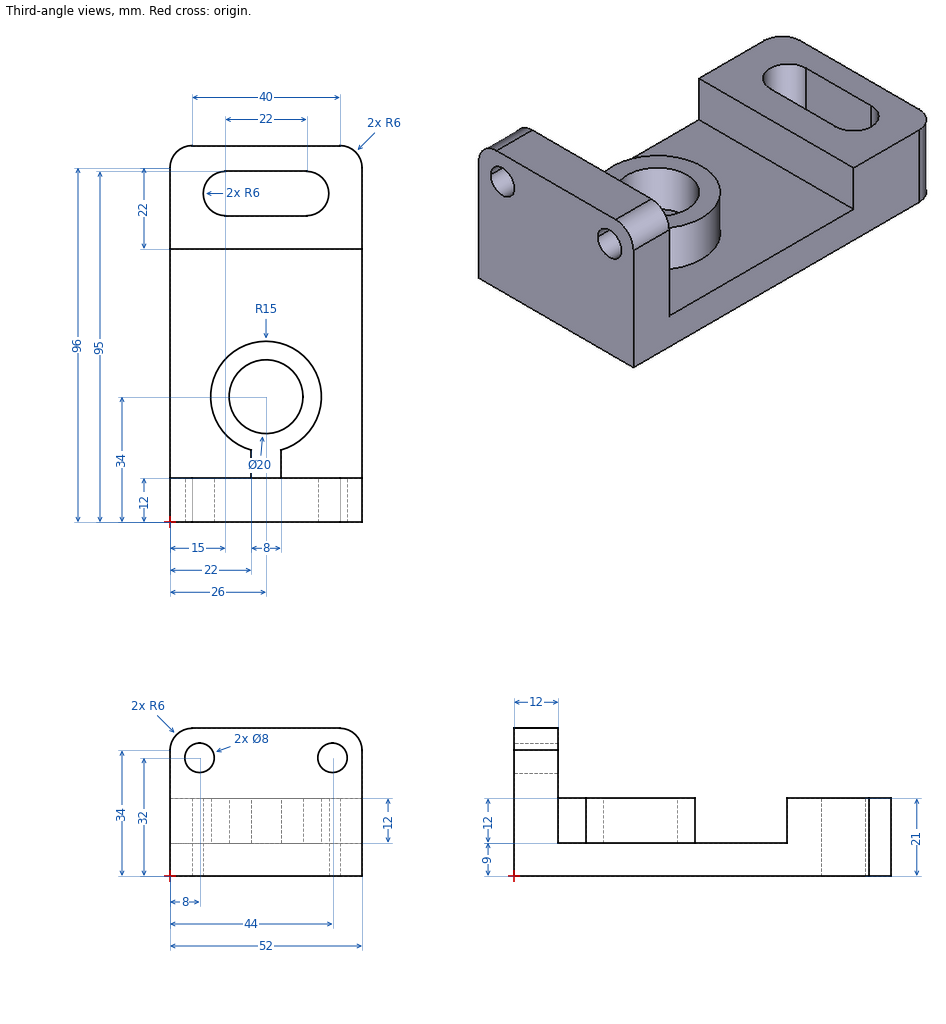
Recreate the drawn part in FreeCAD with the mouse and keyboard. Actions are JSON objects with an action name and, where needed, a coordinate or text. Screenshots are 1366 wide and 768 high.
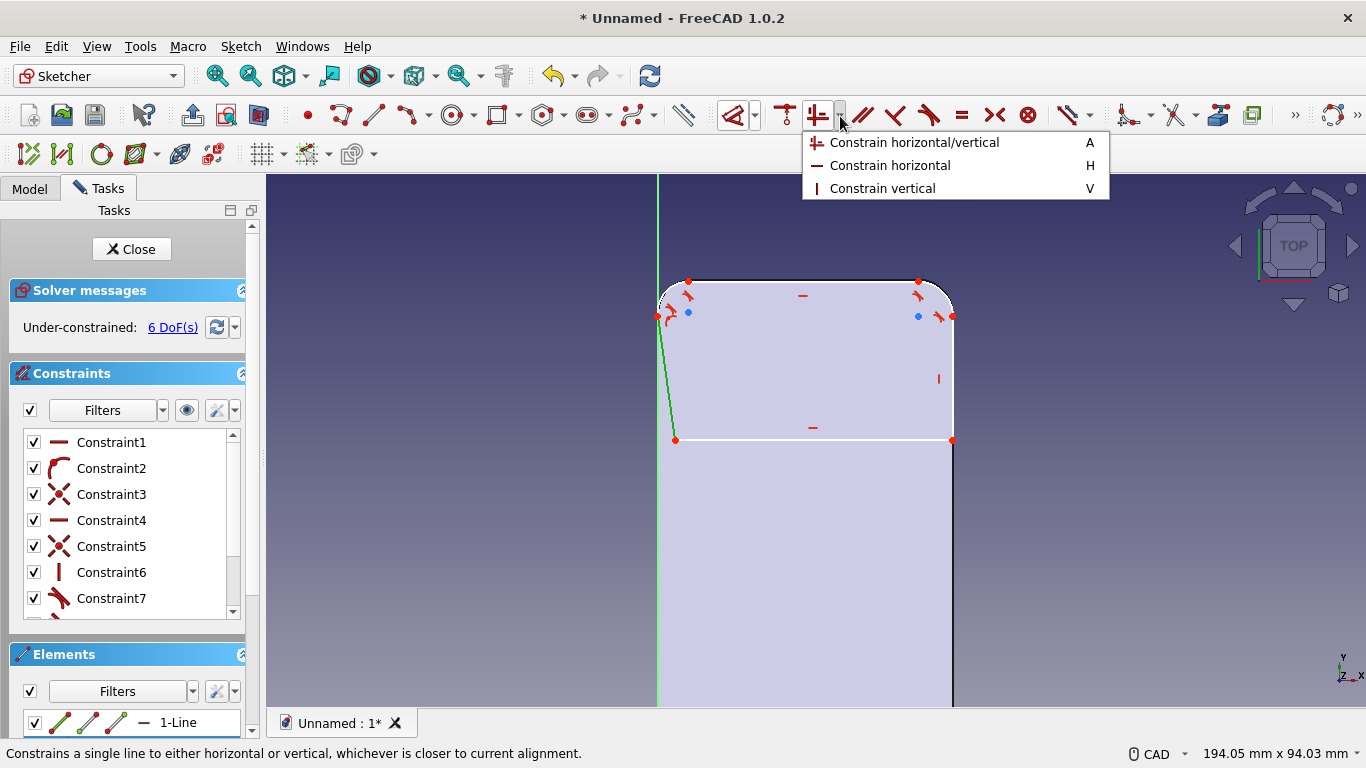
{"action": "left_click", "coordinate": [956, 188]}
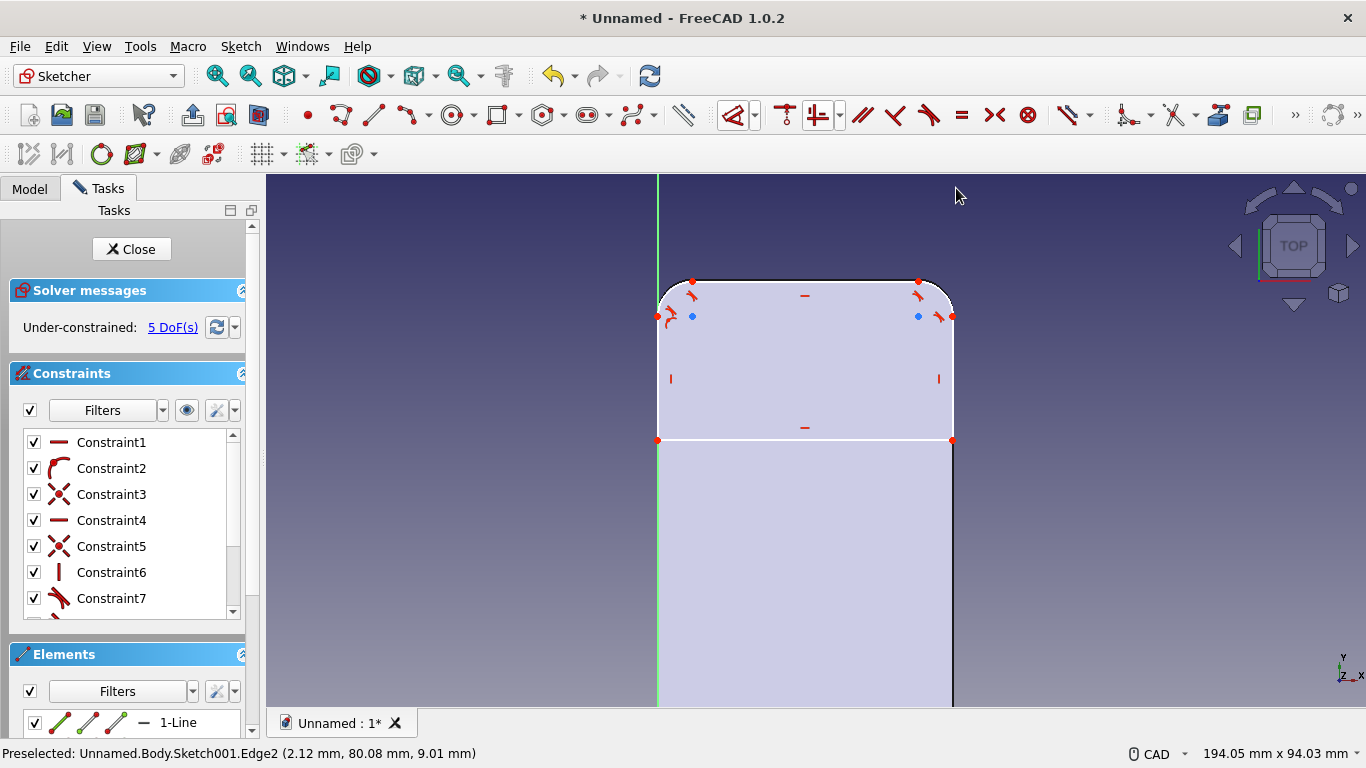
{"action": "left_click", "coordinate": [677, 286]}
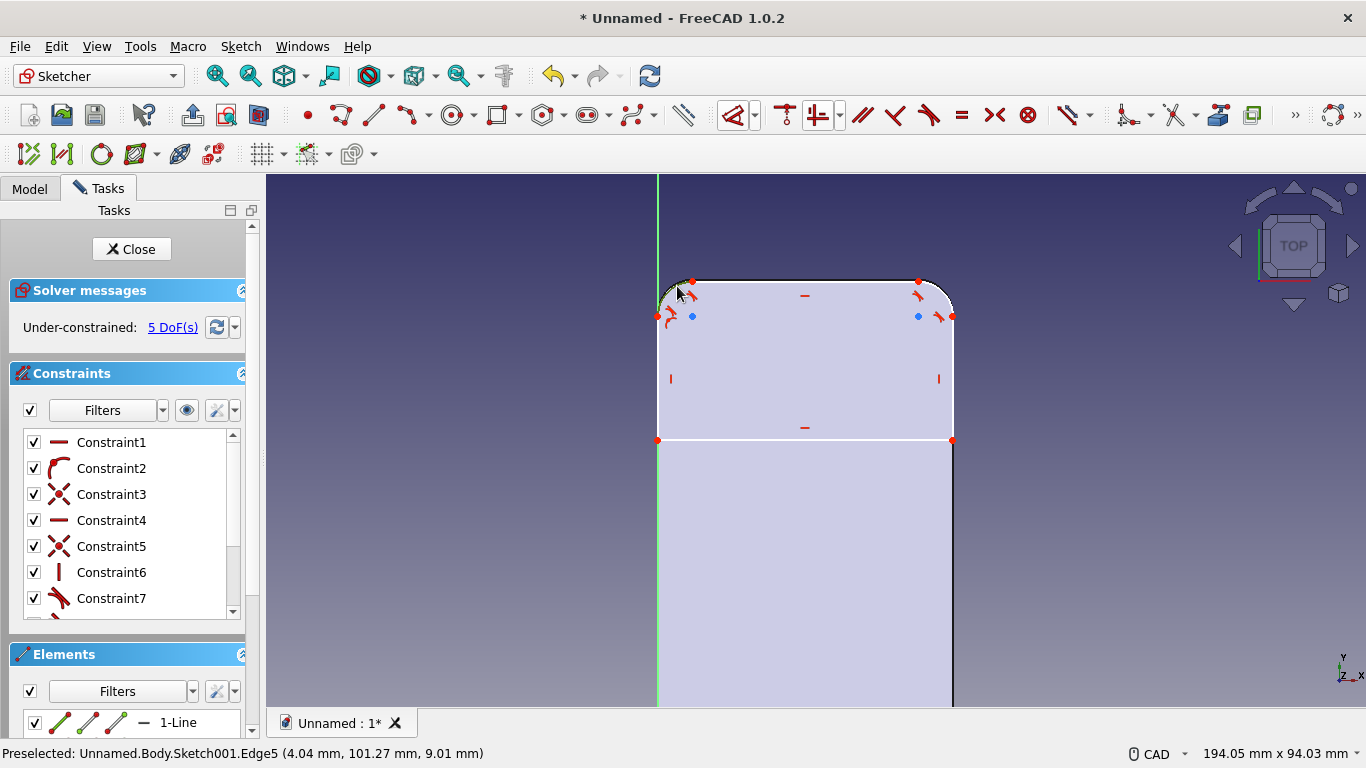
{"action": "left_click", "coordinate": [949, 301]}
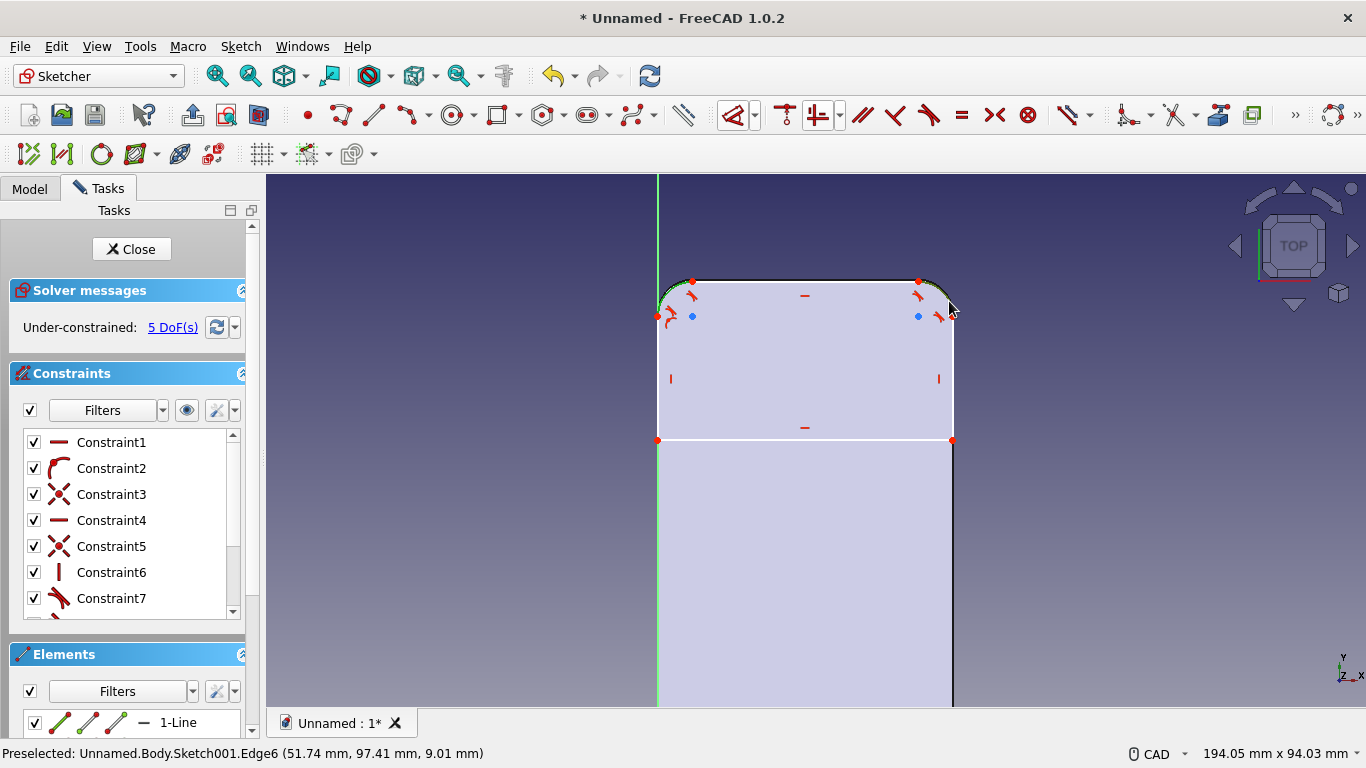
{"action": "left_click", "coordinate": [962, 116]}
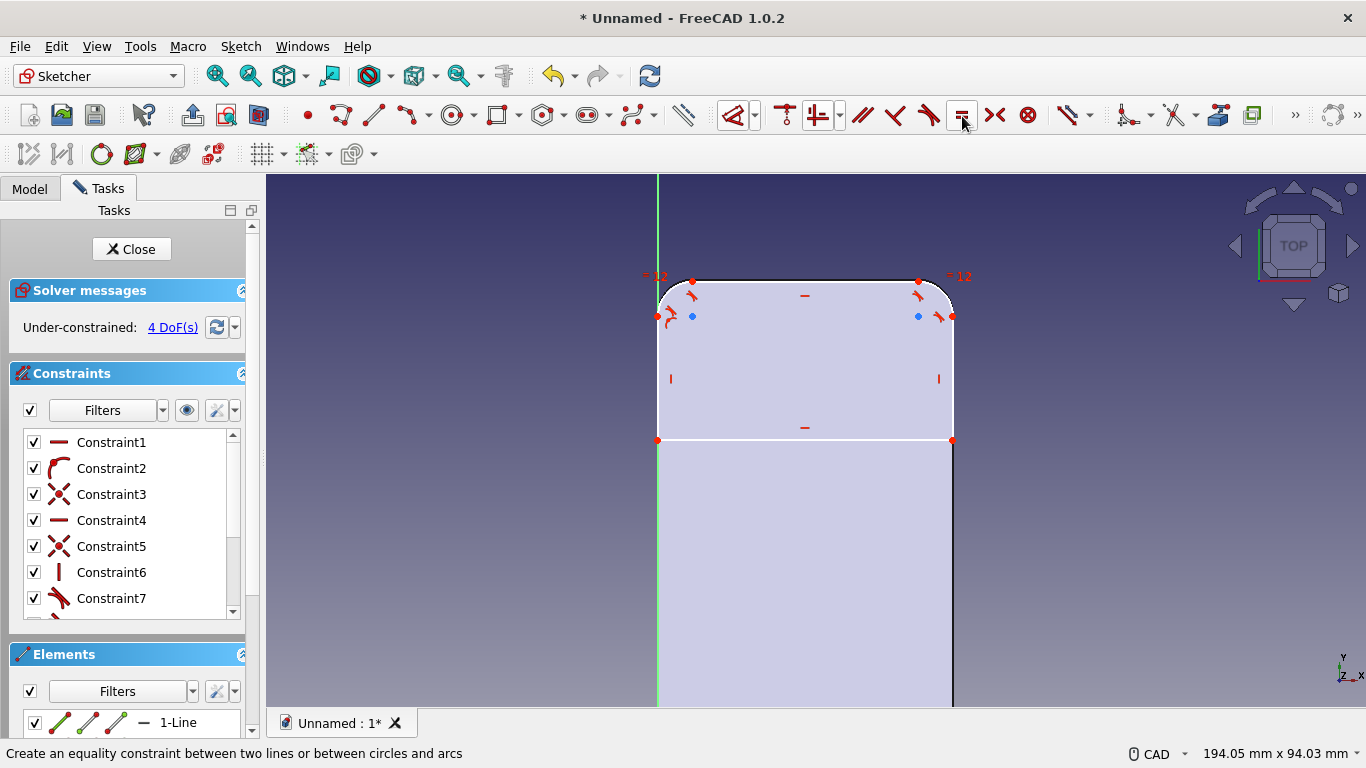
{"action": "left_click", "coordinate": [677, 286]}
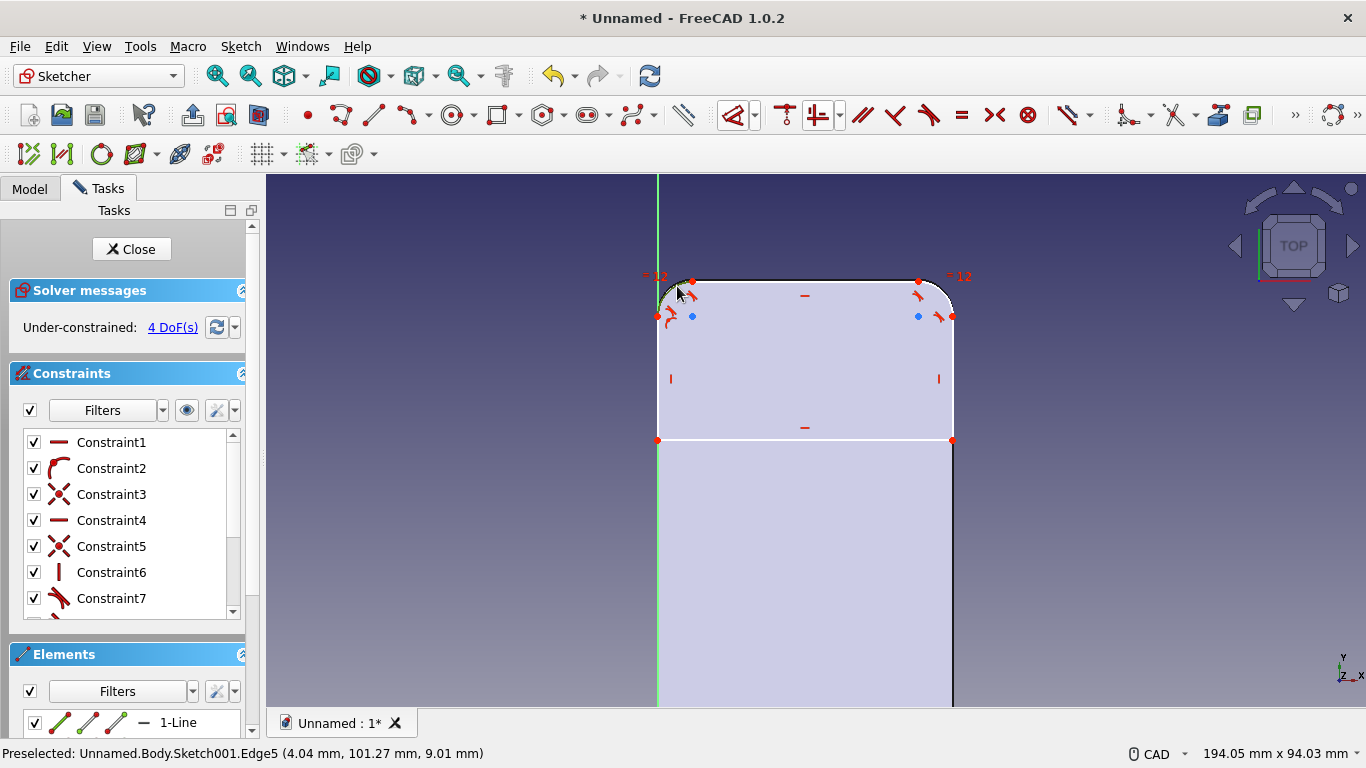
{"action": "key", "text": "k r"}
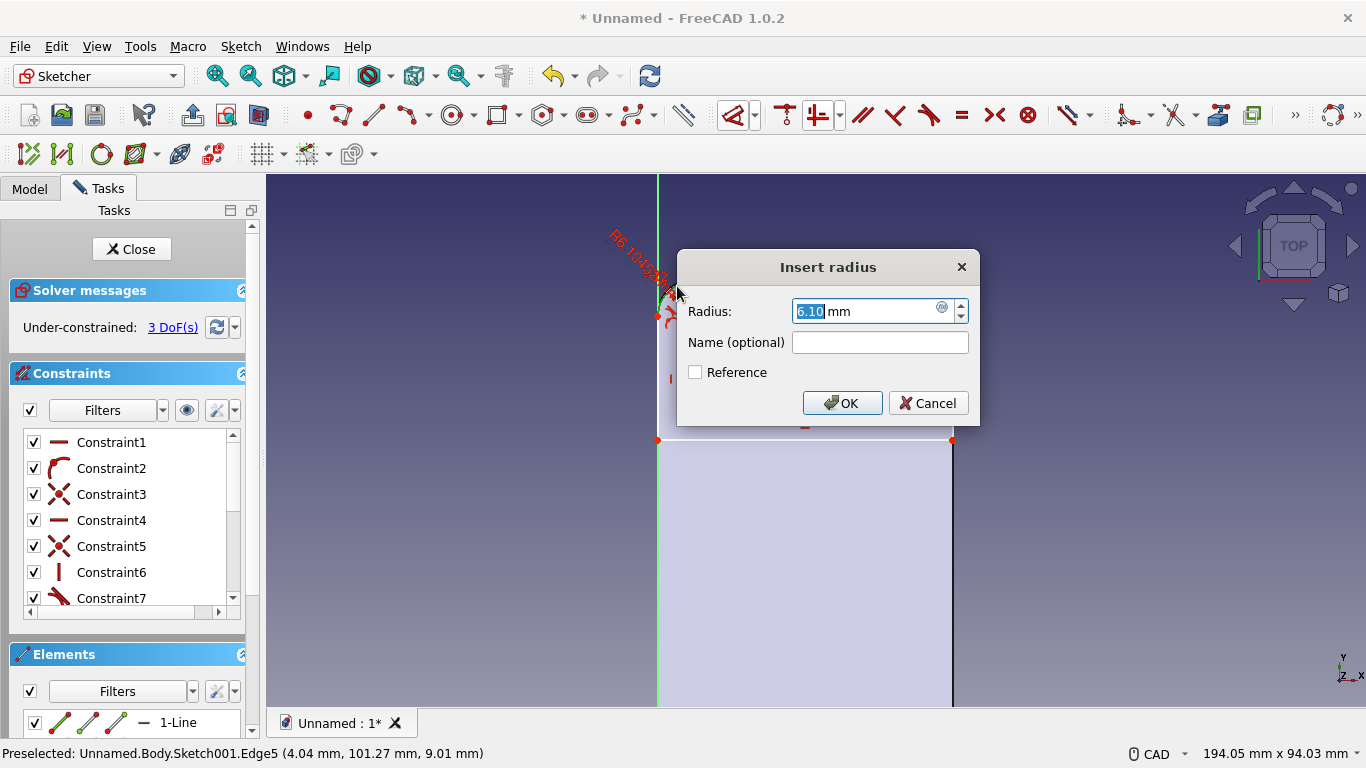
{"action": "type", "text": "6"}
{"action": "key", "text": "Return"}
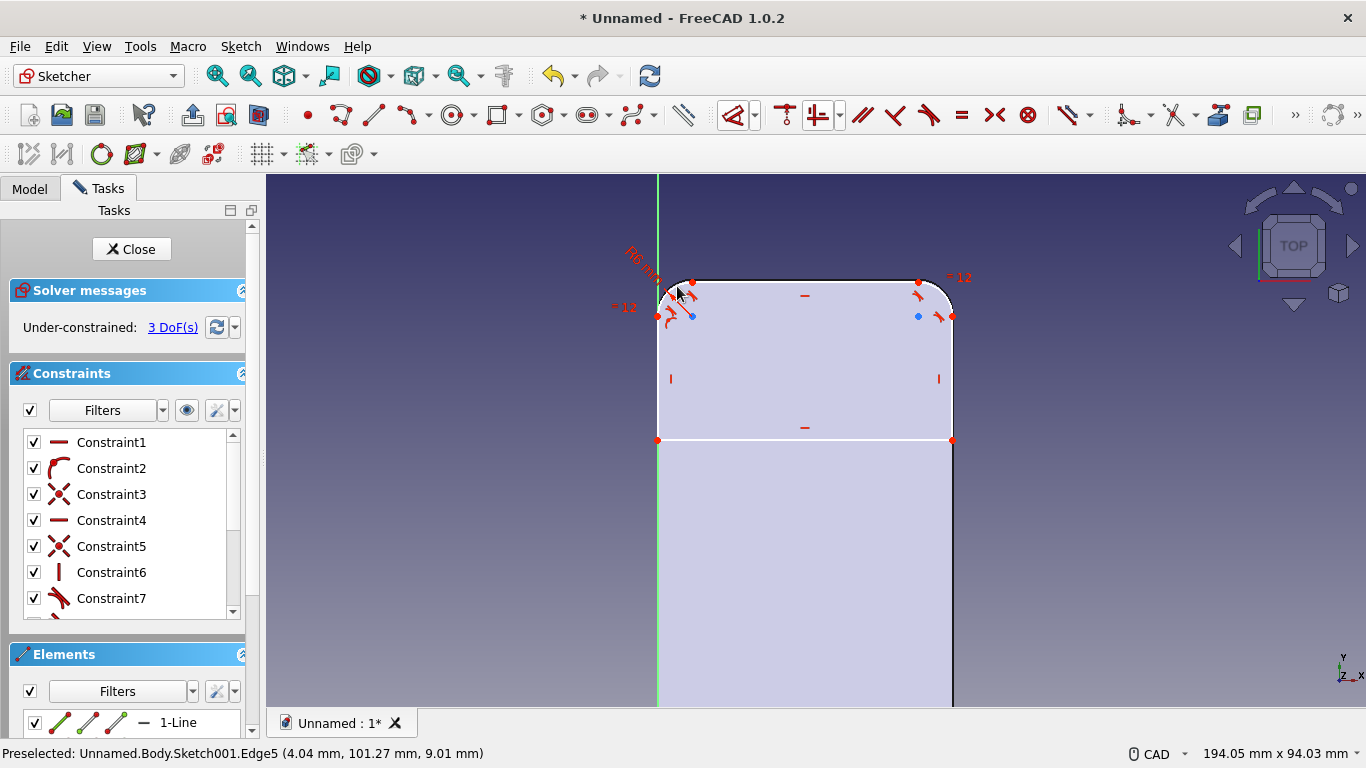
{"action": "left_click", "coordinate": [850, 282]}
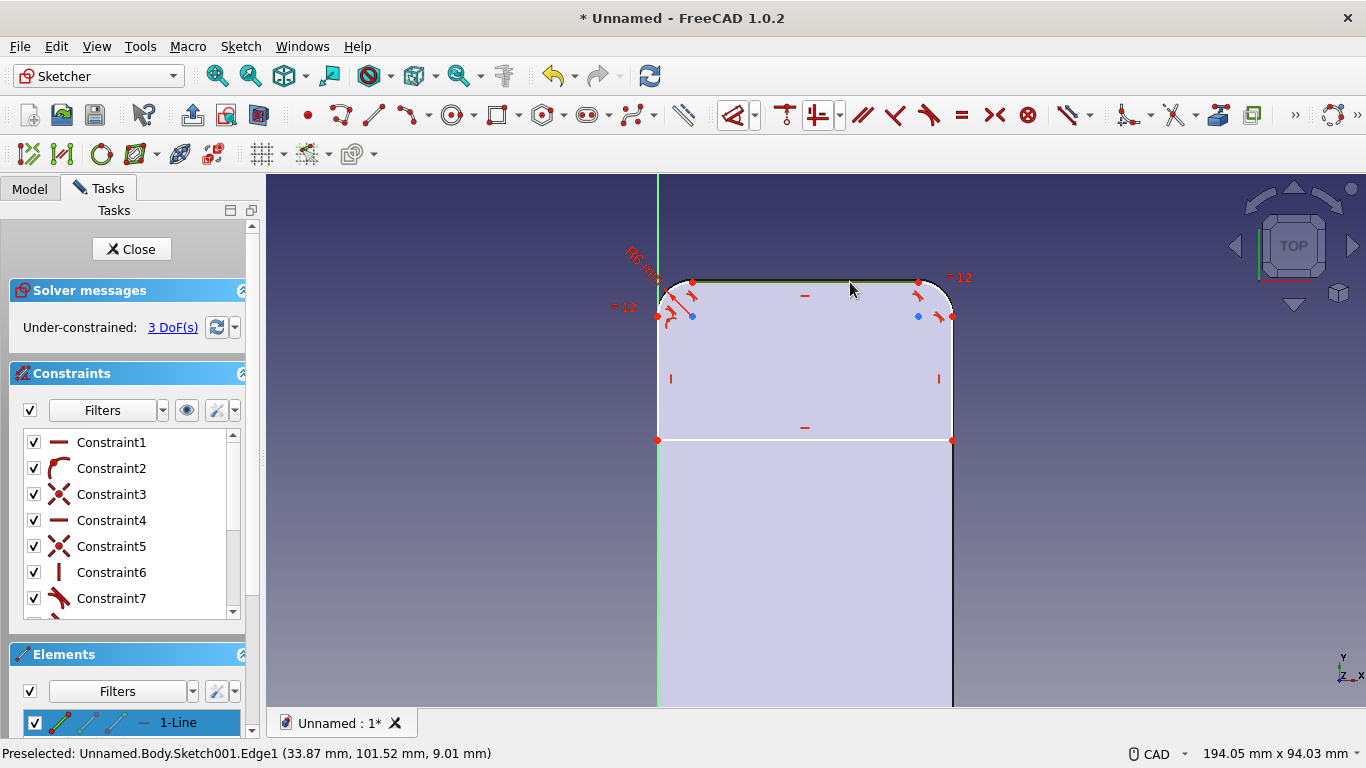
{"action": "left_click", "coordinate": [754, 116]}